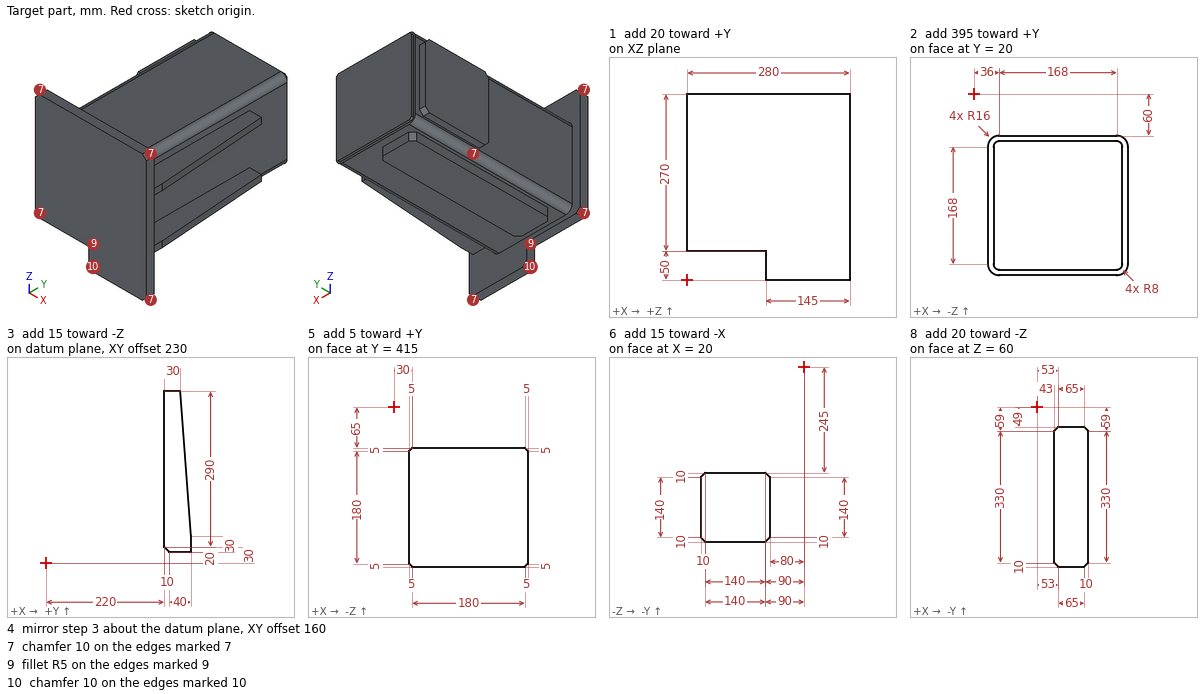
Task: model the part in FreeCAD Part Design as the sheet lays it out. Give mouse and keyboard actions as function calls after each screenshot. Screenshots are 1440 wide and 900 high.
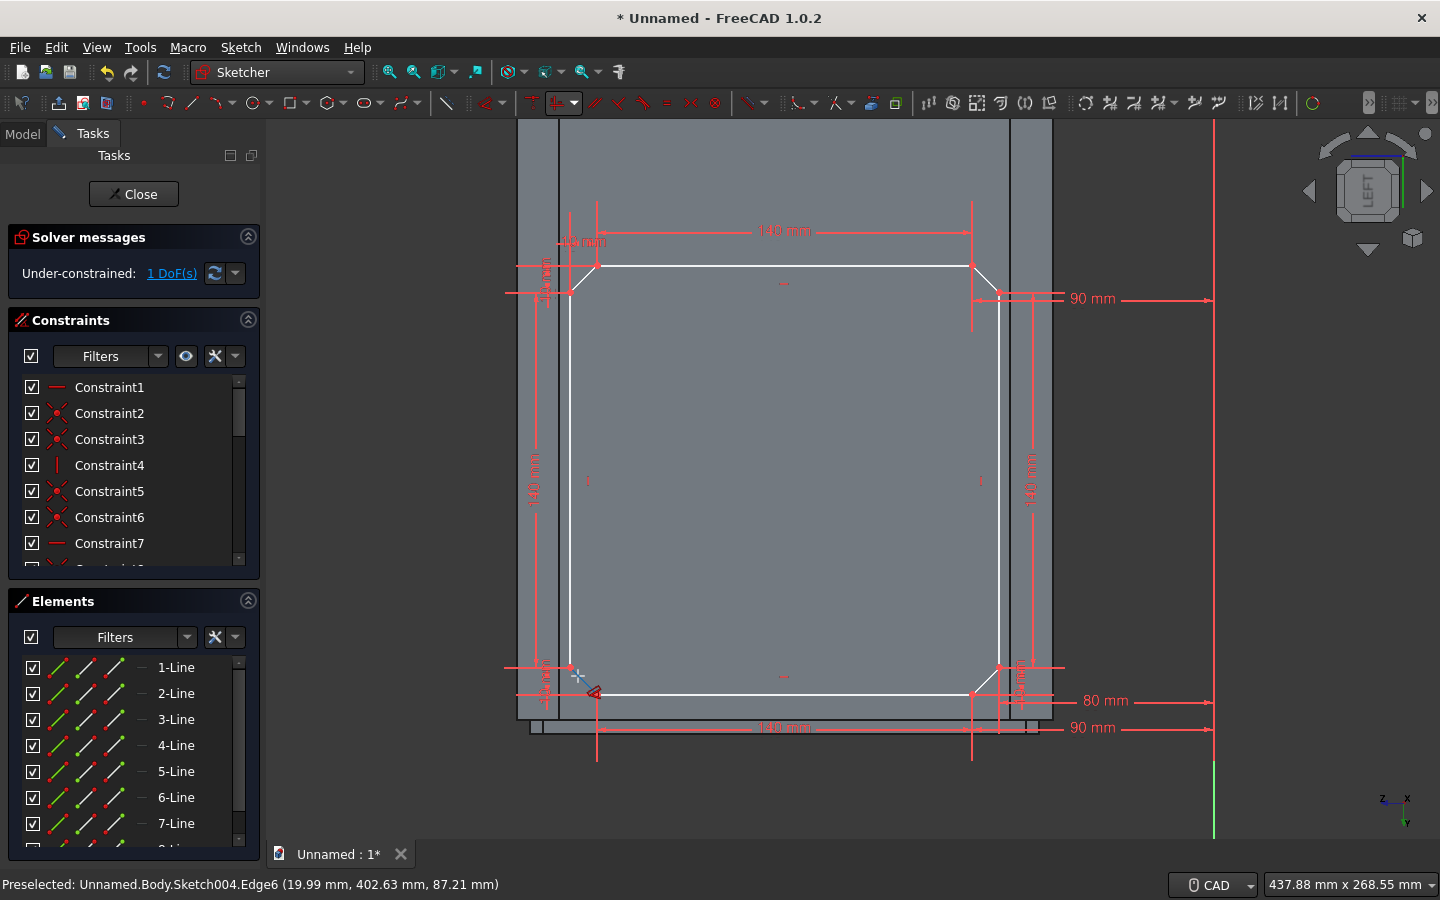
click(972, 266)
click(1248, 206)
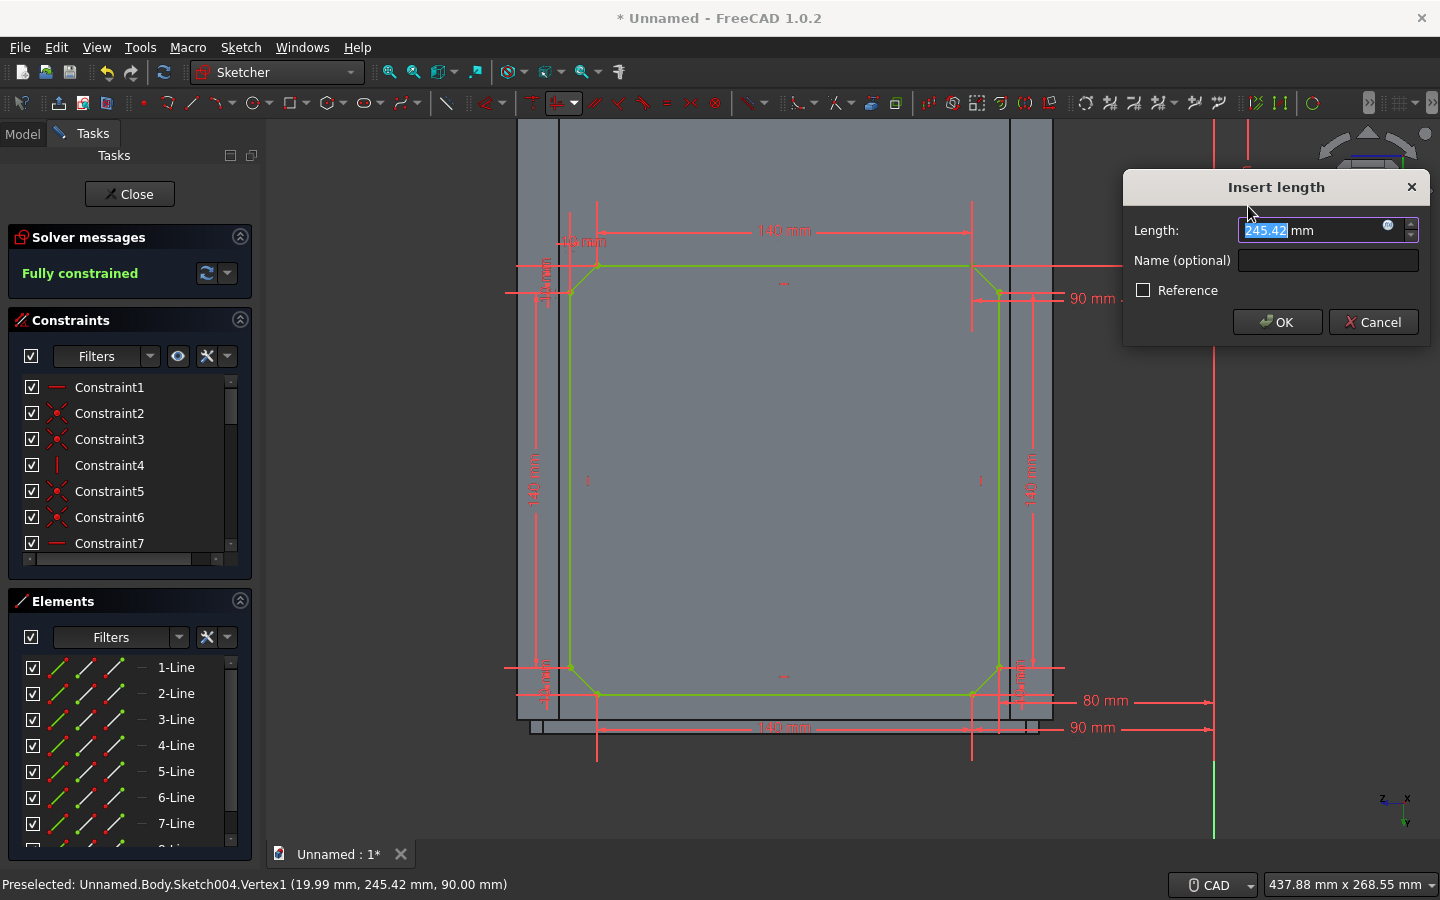
text(245)
key(Return)
key(Escape)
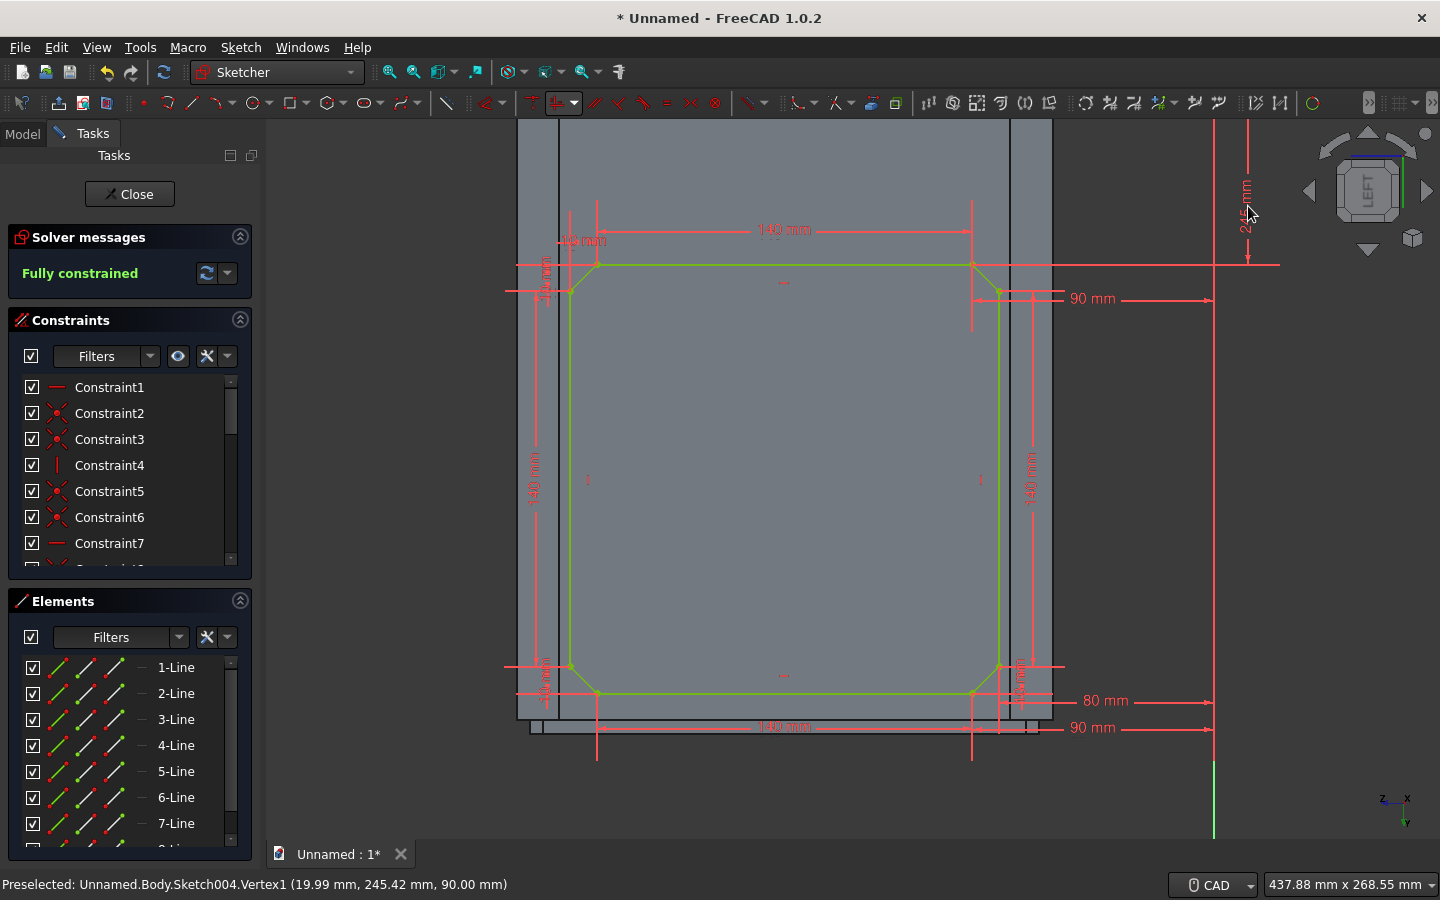
click(130, 194)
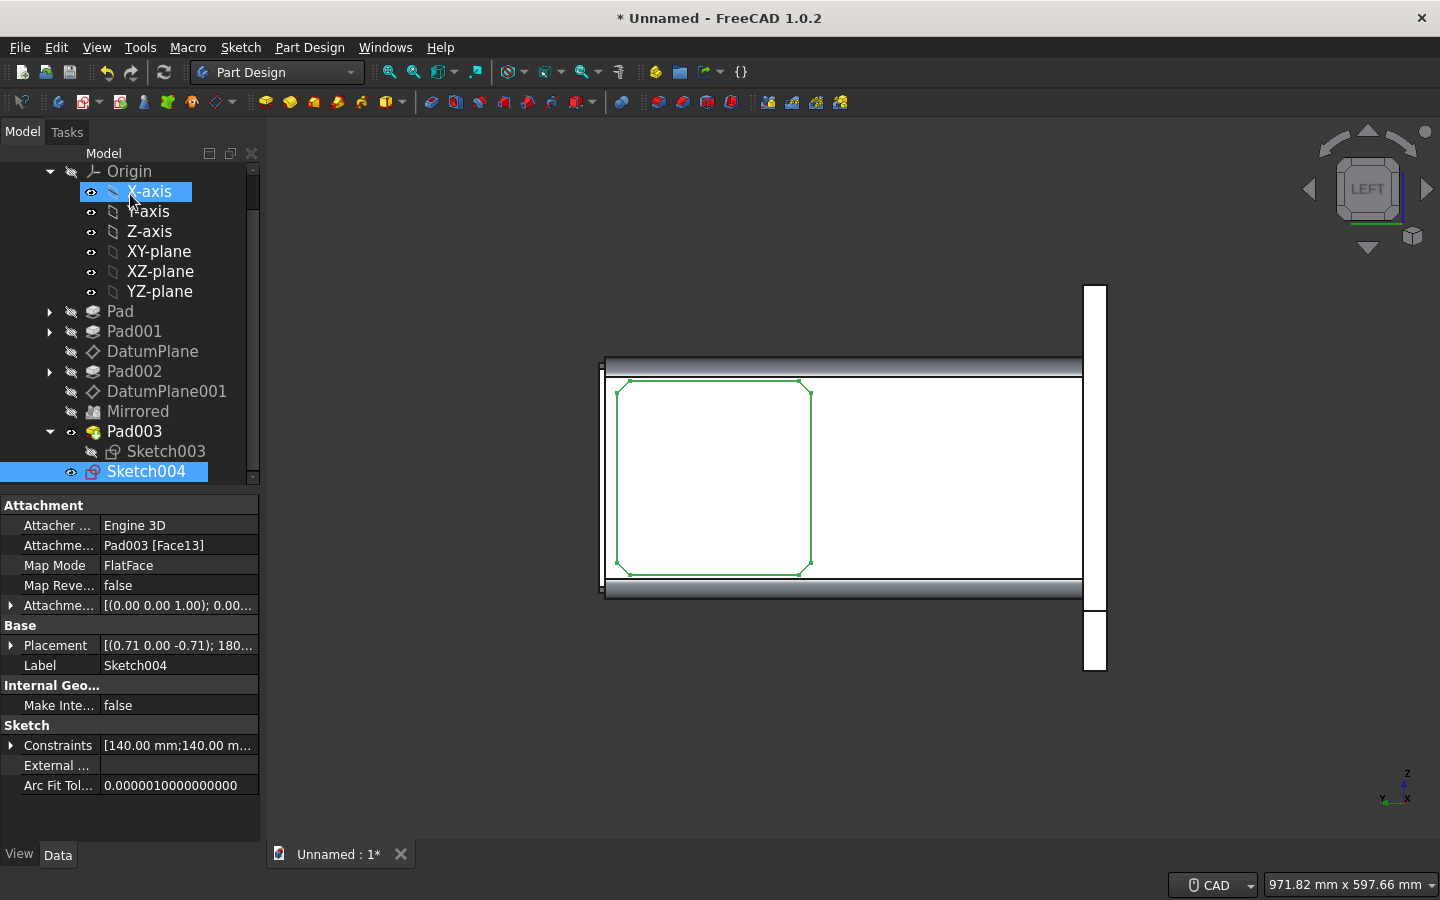
click(266, 102)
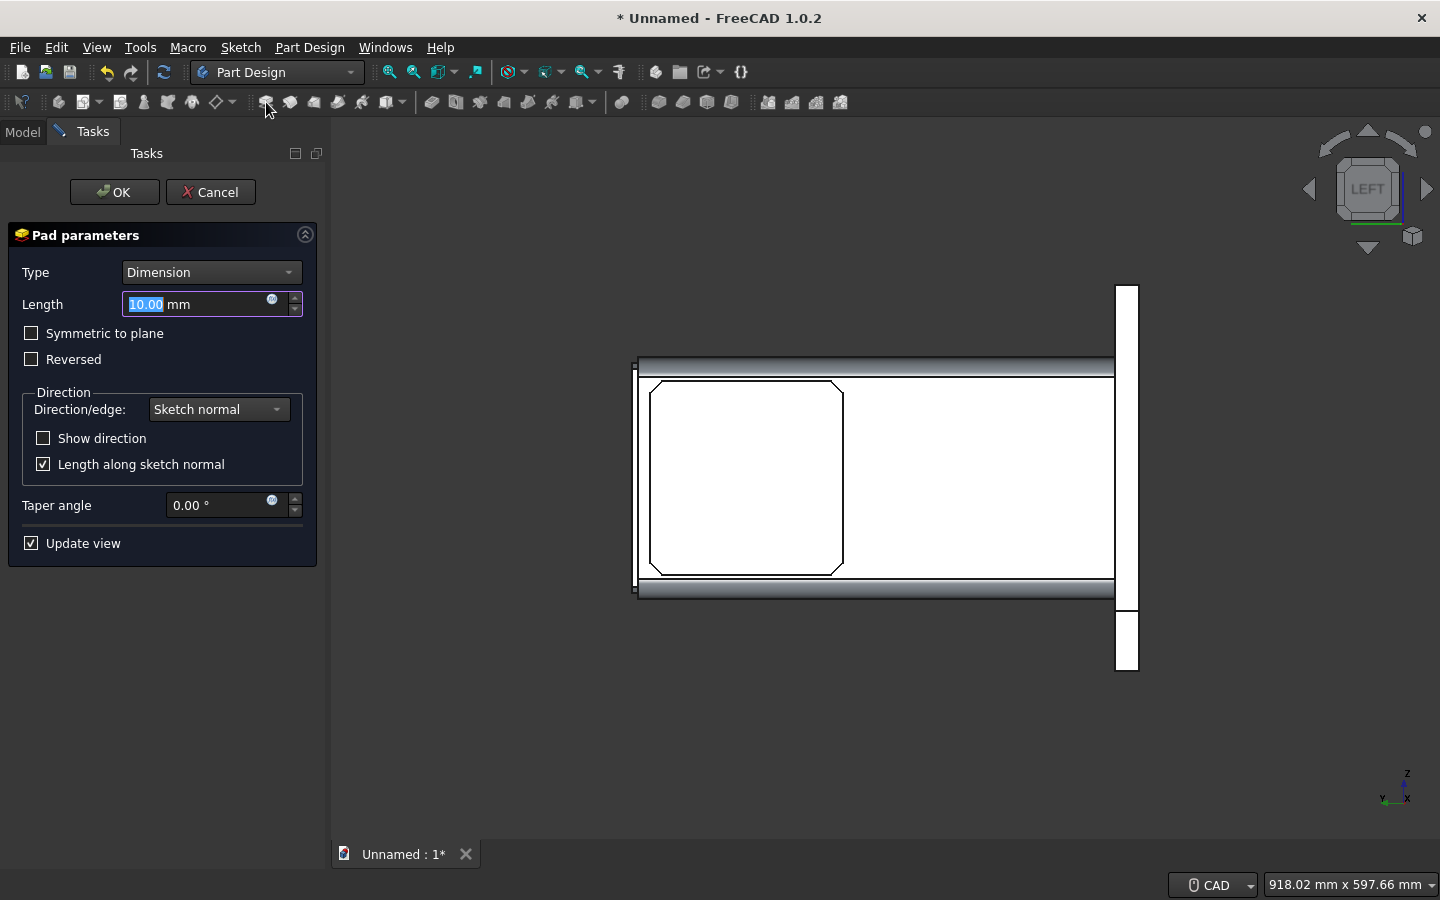
text(15)
key(Tab)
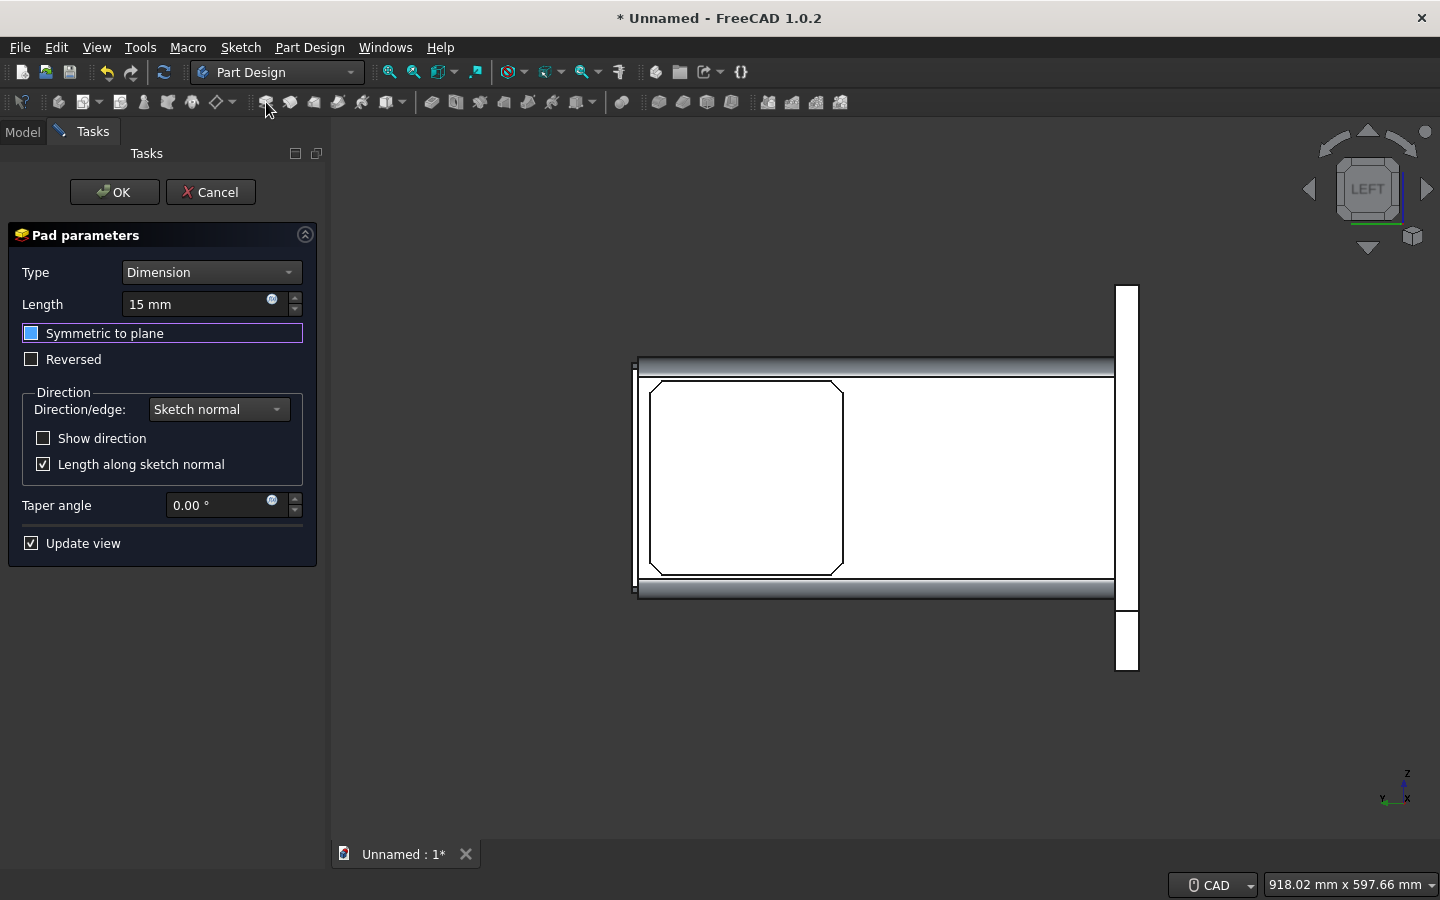
click(115, 192)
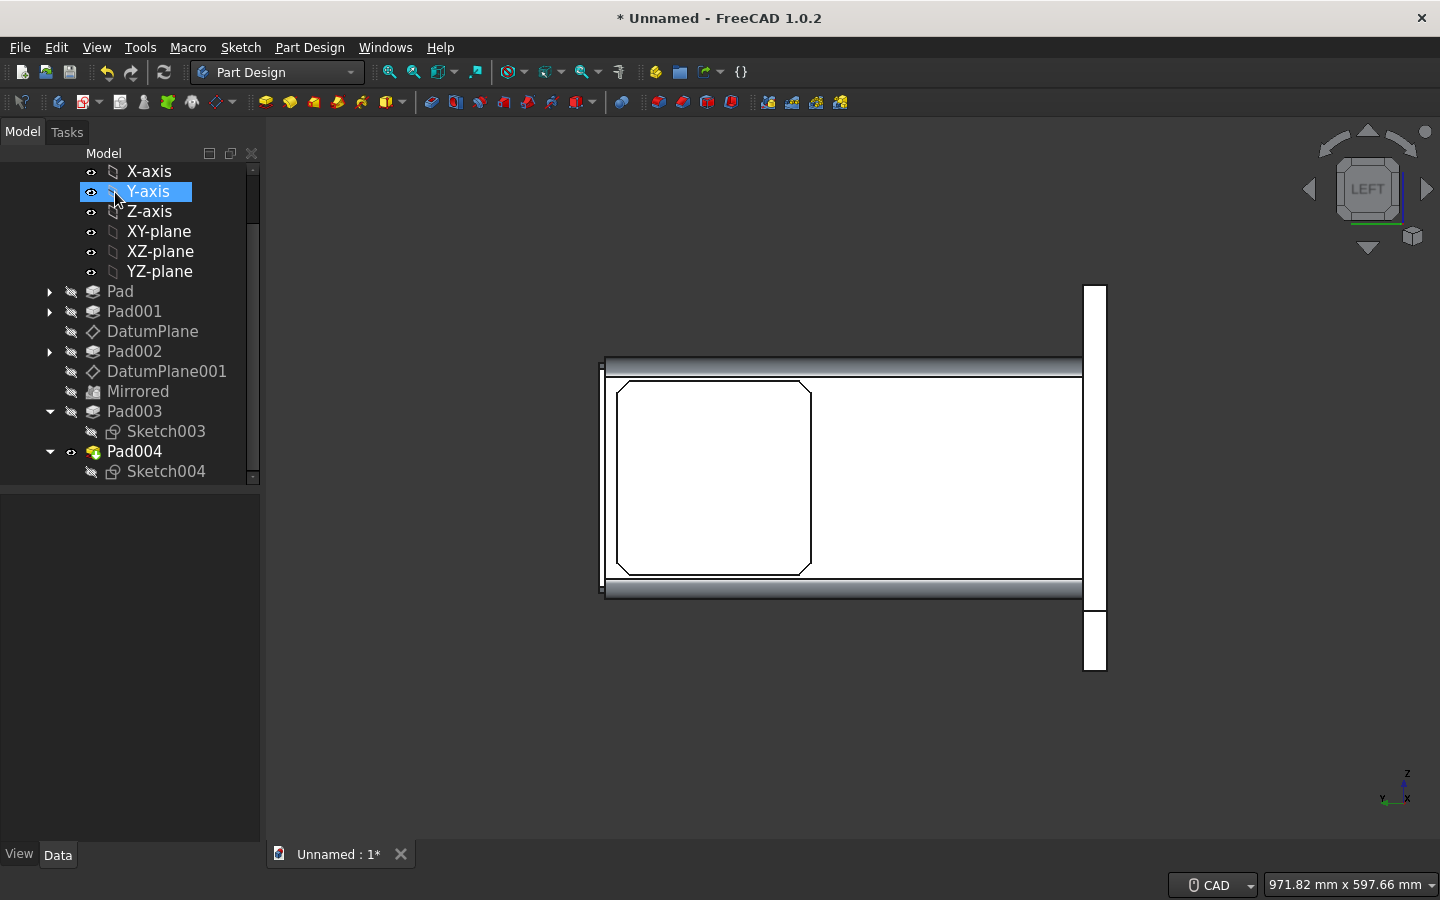
click(1095, 284)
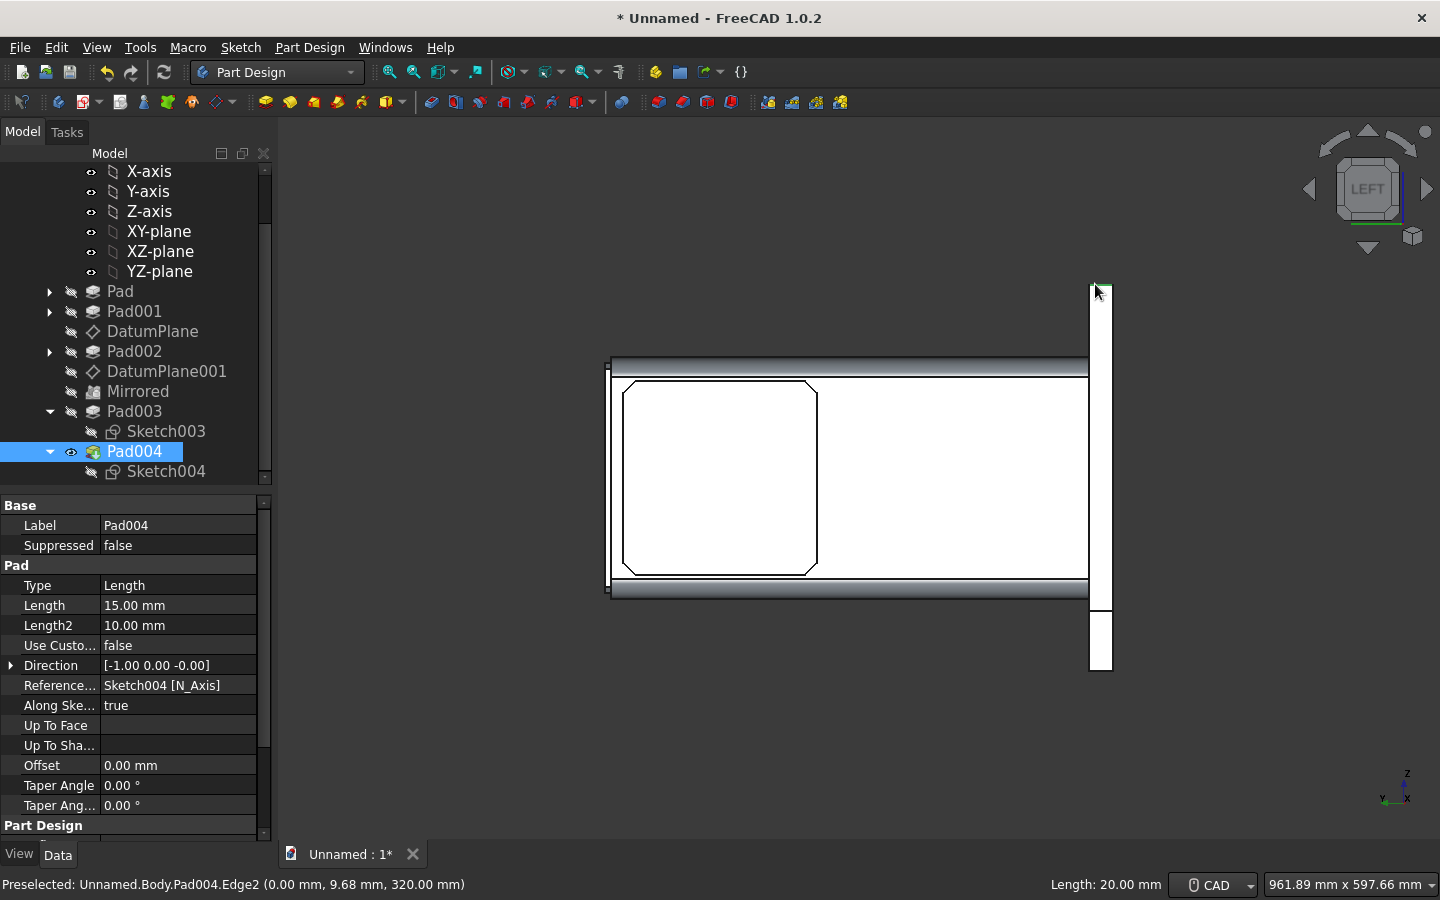
click(1101, 610, ctrl)